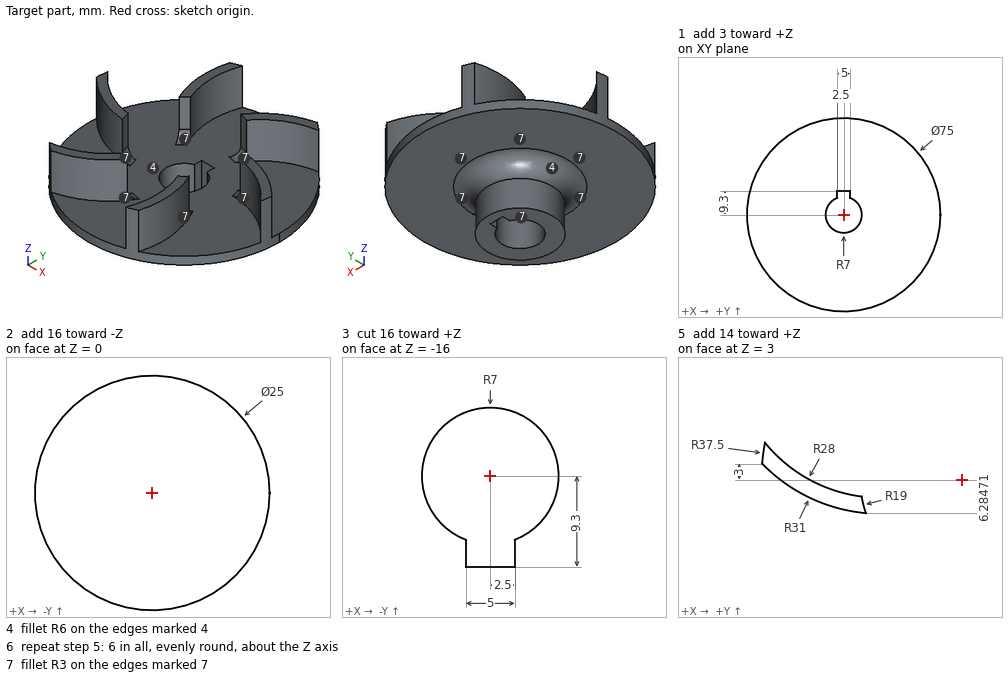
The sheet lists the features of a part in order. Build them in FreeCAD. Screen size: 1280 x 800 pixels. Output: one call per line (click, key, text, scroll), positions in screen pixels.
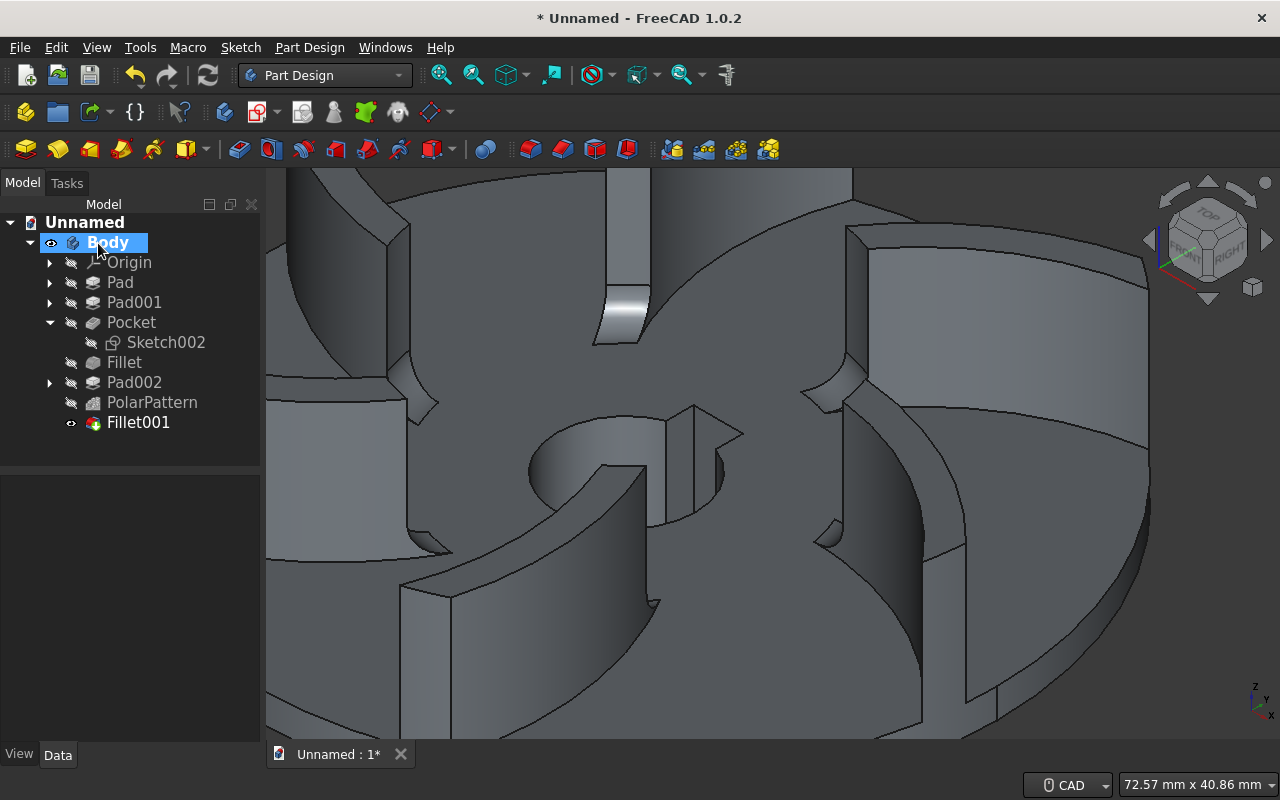
click(442, 76)